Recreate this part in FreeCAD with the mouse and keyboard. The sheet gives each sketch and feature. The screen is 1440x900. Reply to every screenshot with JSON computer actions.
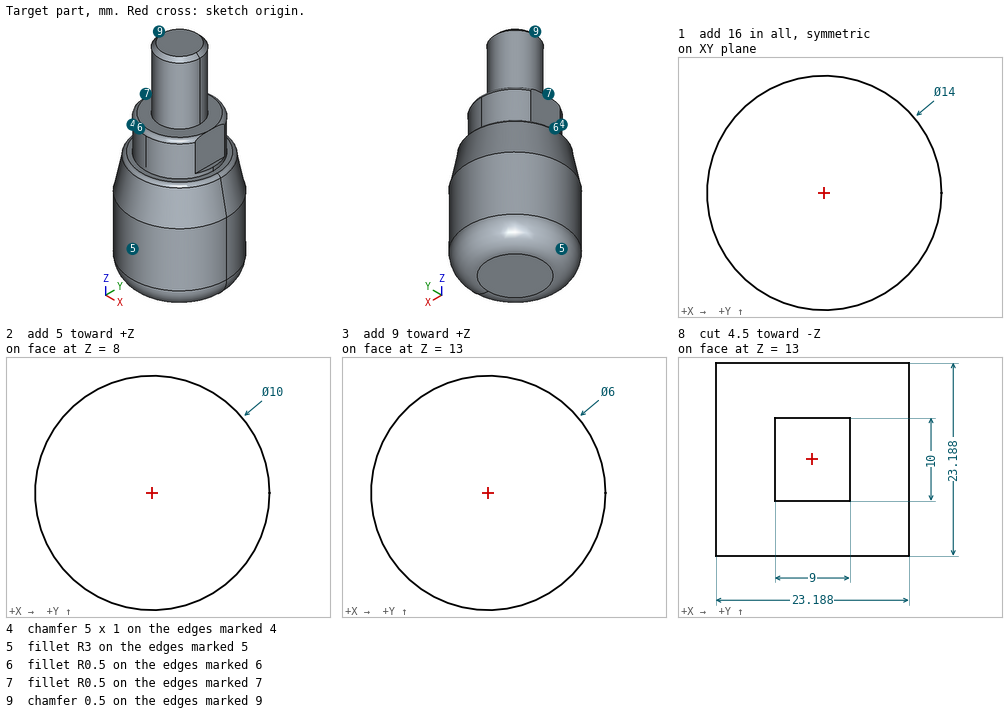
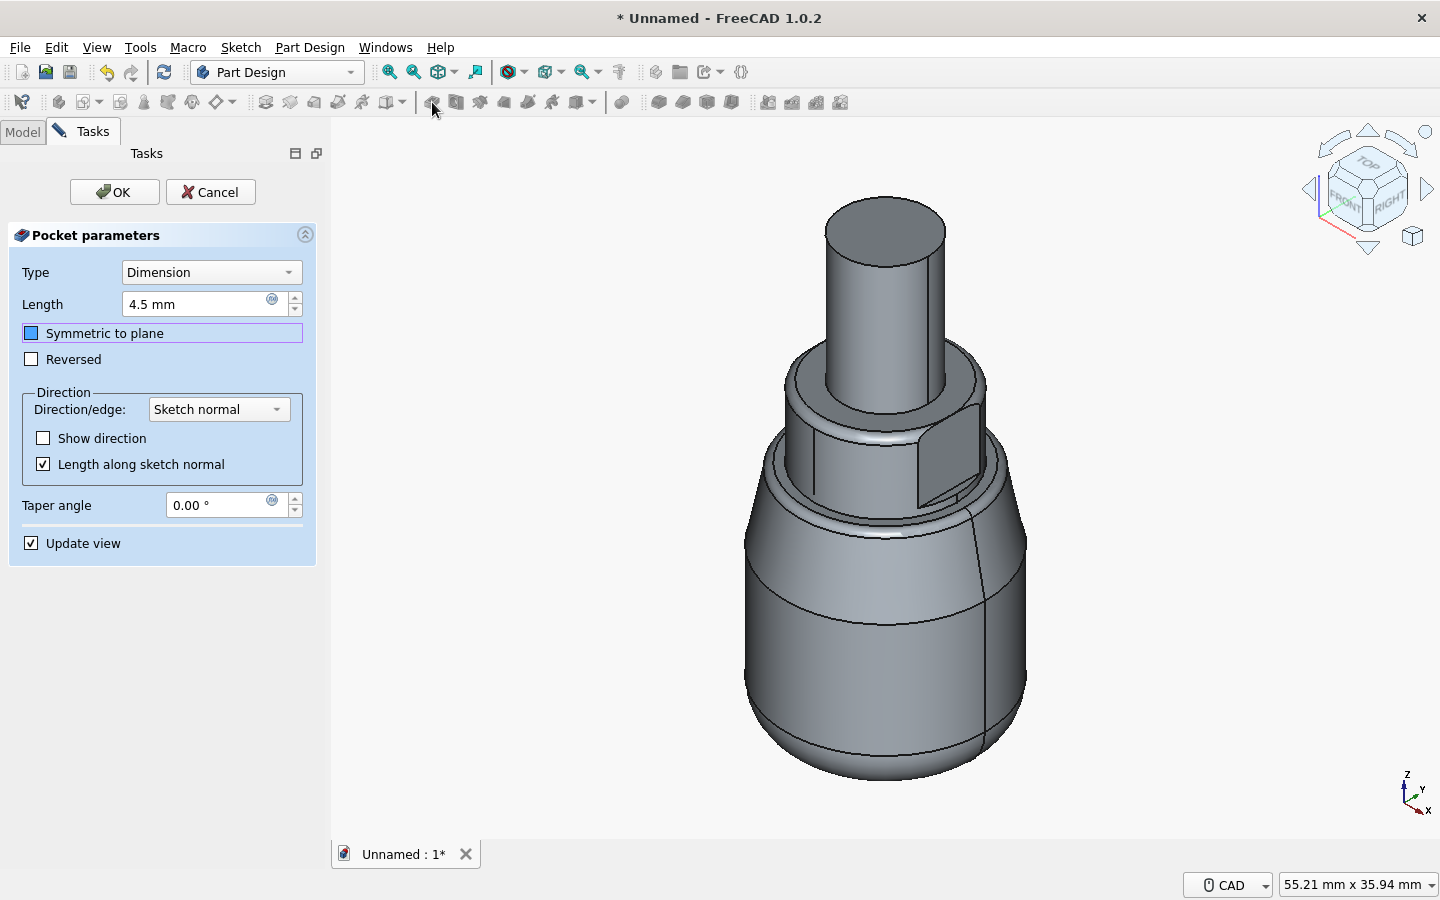
{"action": "left_click", "coordinate": [115, 192]}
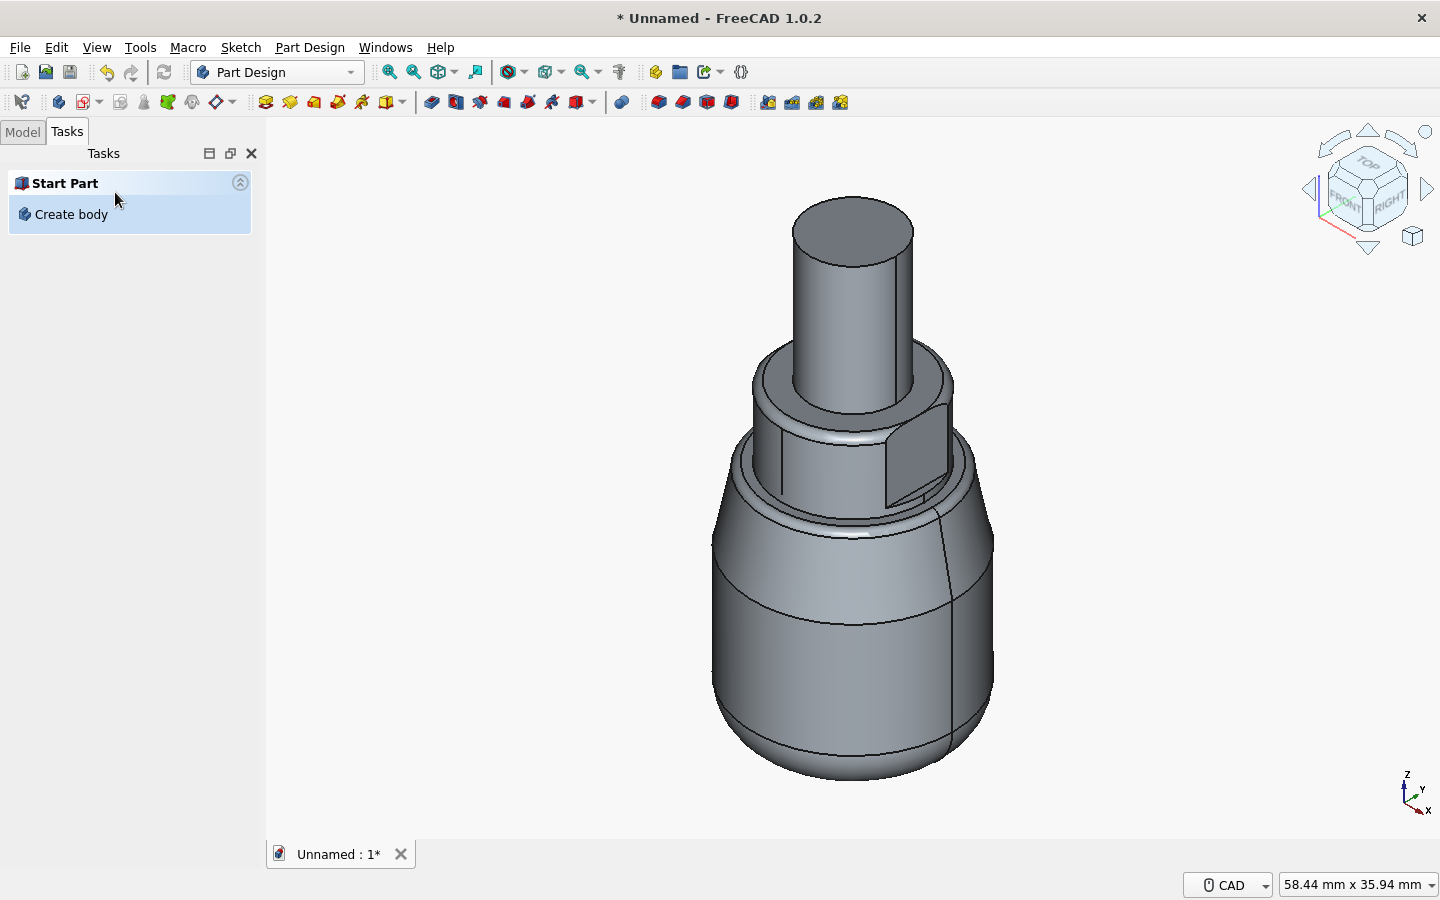
{"action": "key", "text": "v f"}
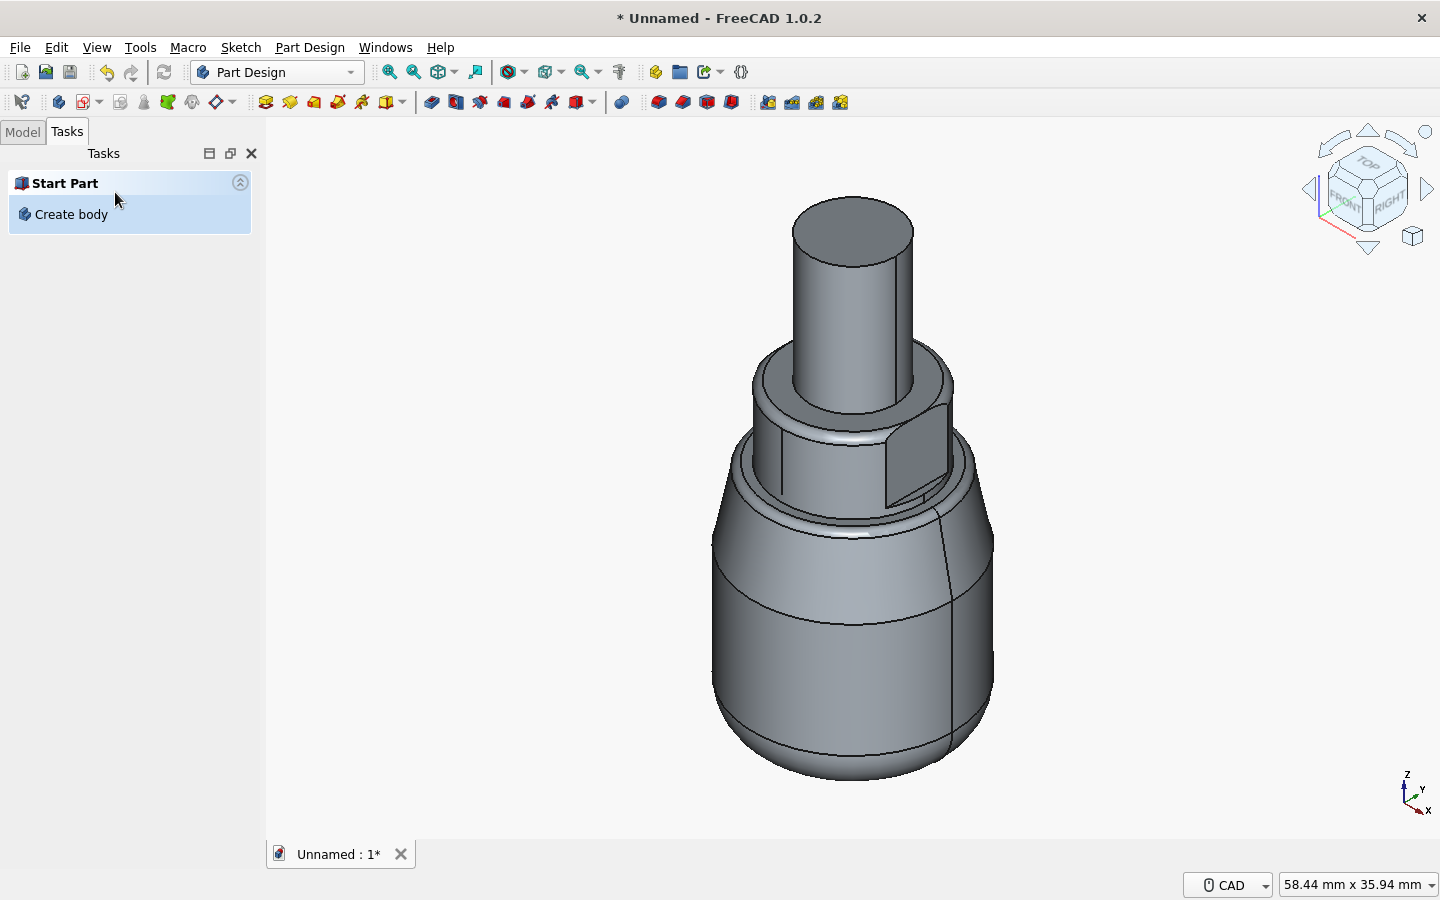
{"action": "left_click", "coordinate": [793, 226]}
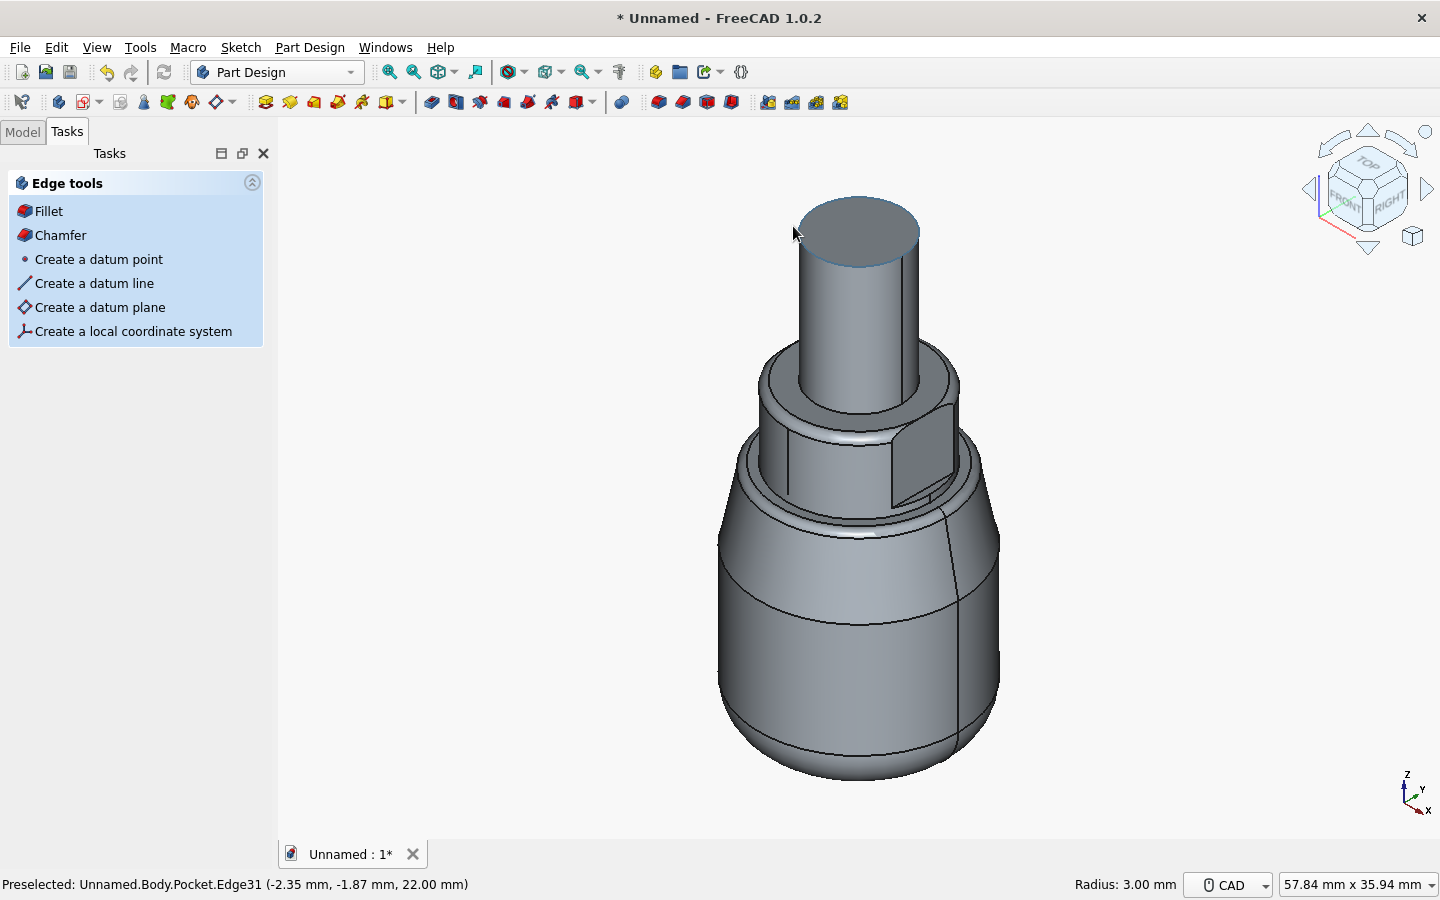
{"action": "left_click", "coordinate": [684, 102]}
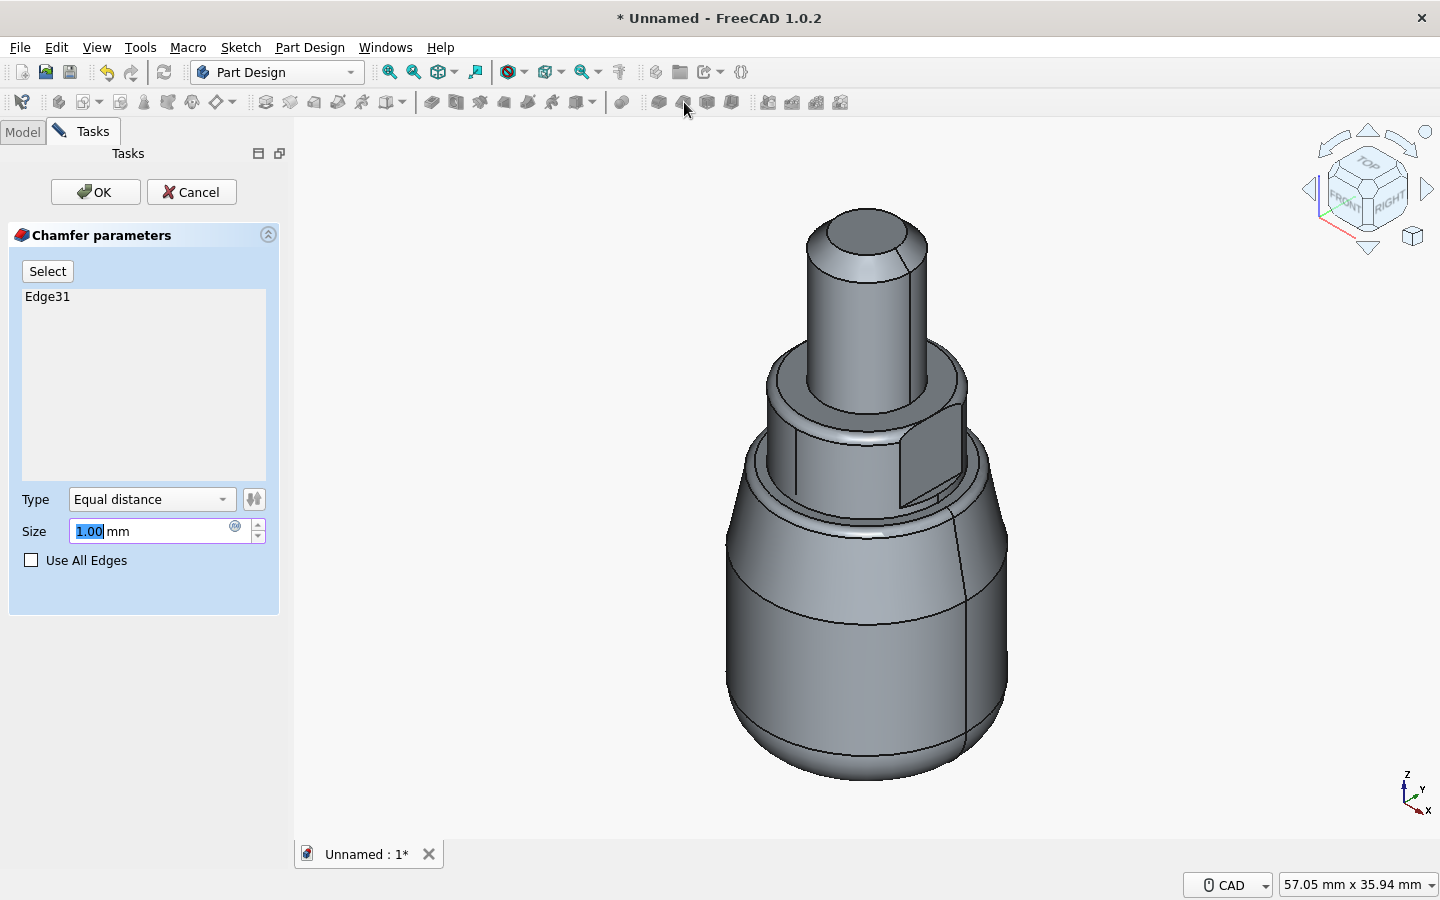
{"action": "type", "text": "0.5"}
{"action": "key", "text": "Tab"}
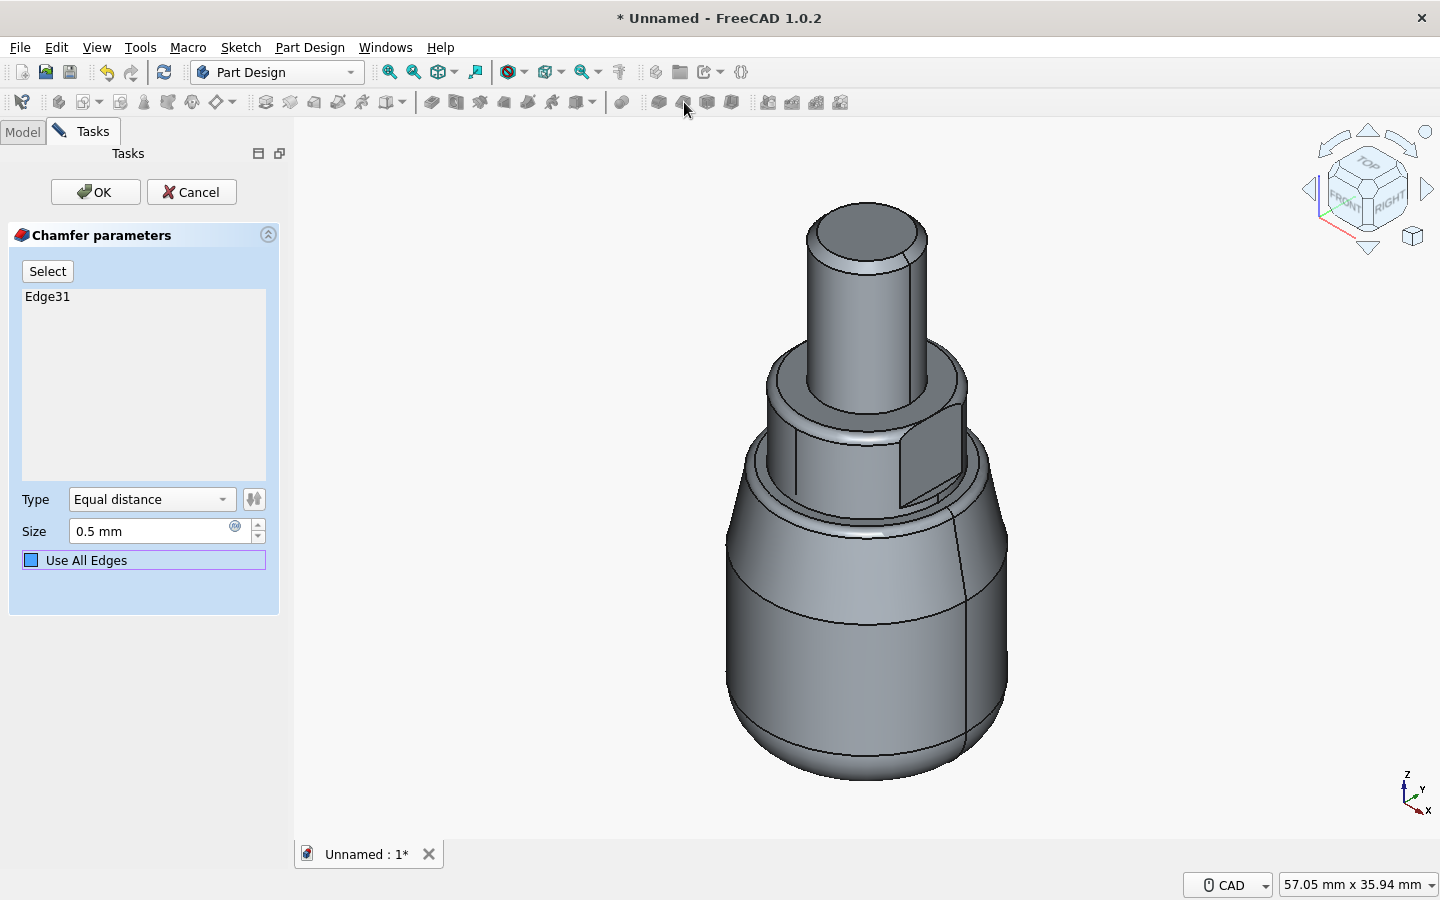
{"action": "left_click", "coordinate": [96, 192]}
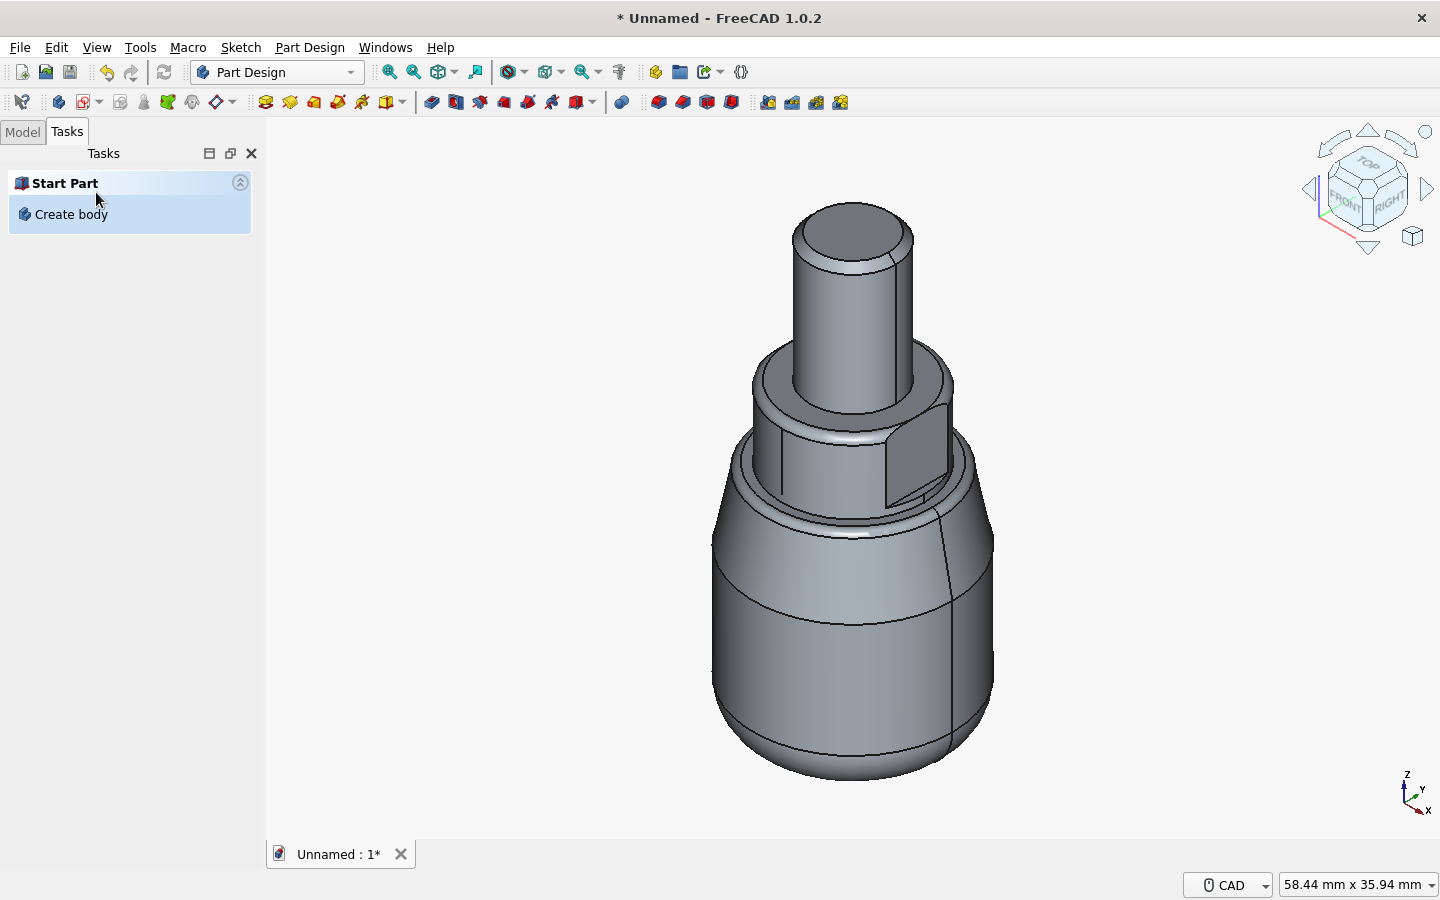
{"action": "key", "text": "v f"}